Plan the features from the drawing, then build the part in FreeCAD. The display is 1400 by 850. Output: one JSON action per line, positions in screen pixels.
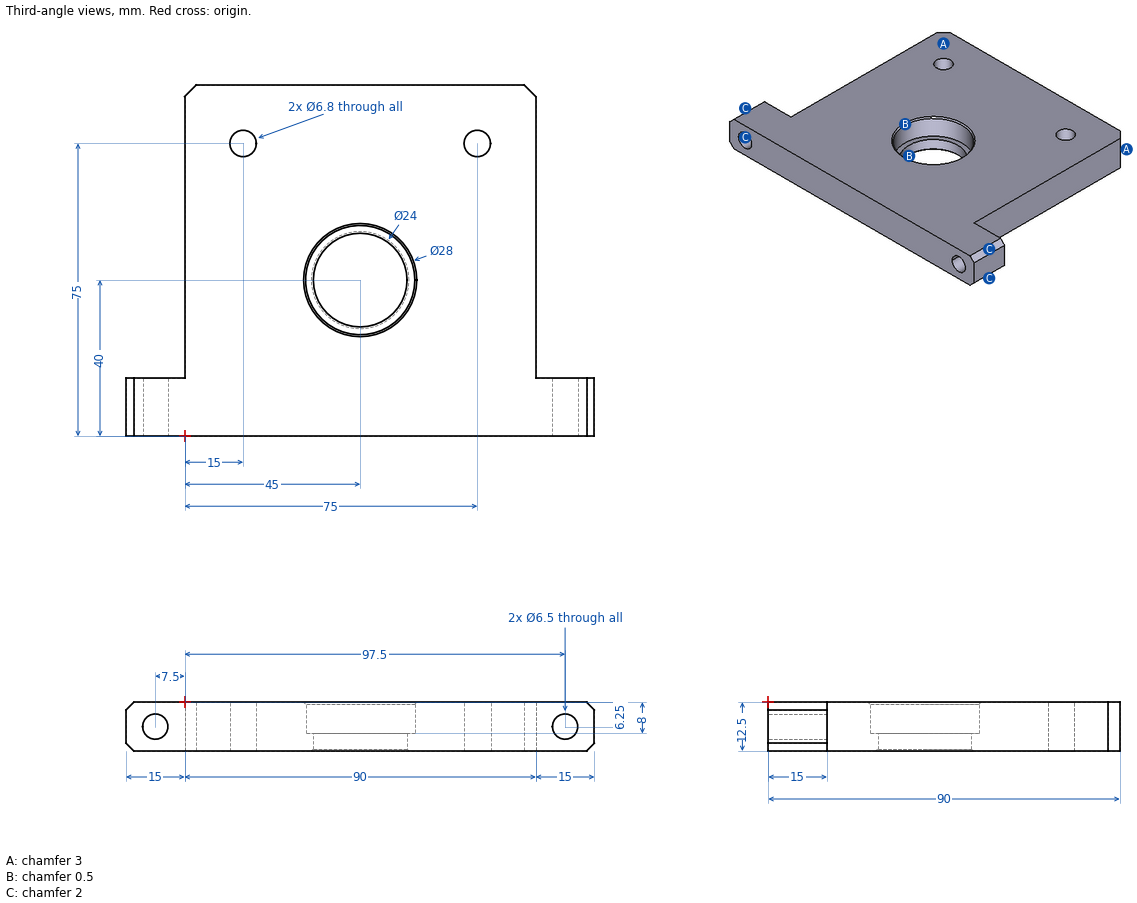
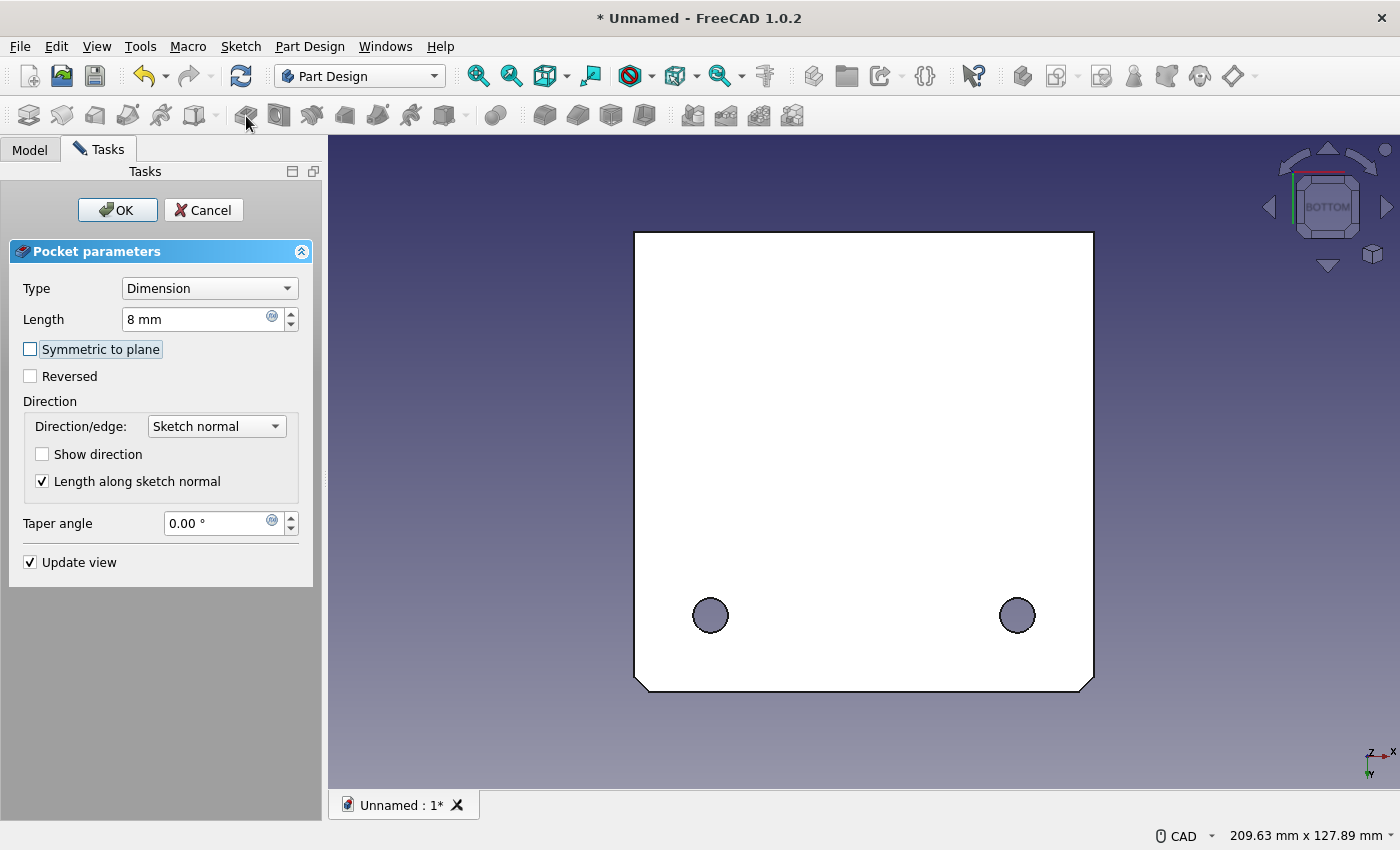
{"action": "left_click", "coordinate": [118, 210]}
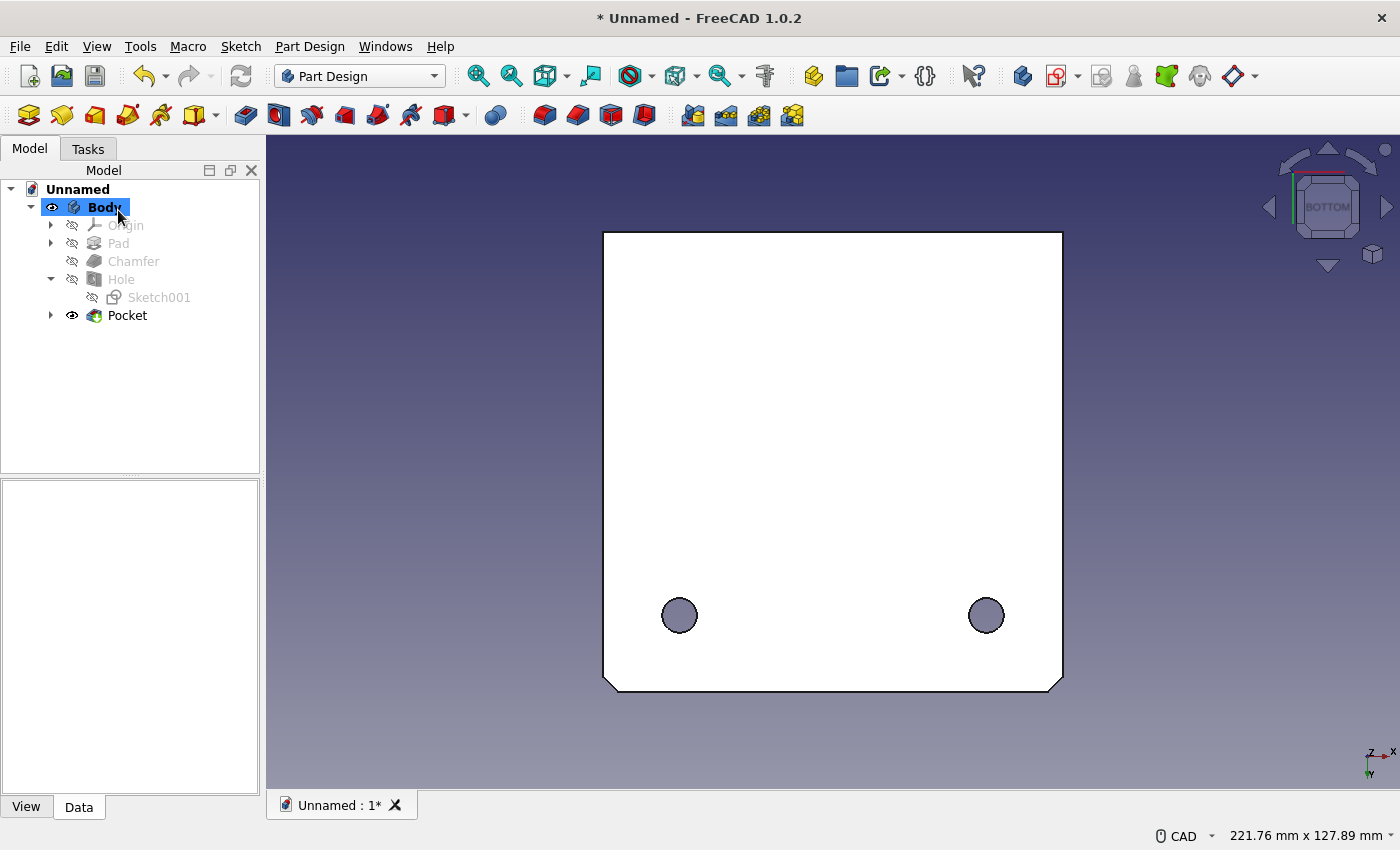
{"action": "key", "text": "0"}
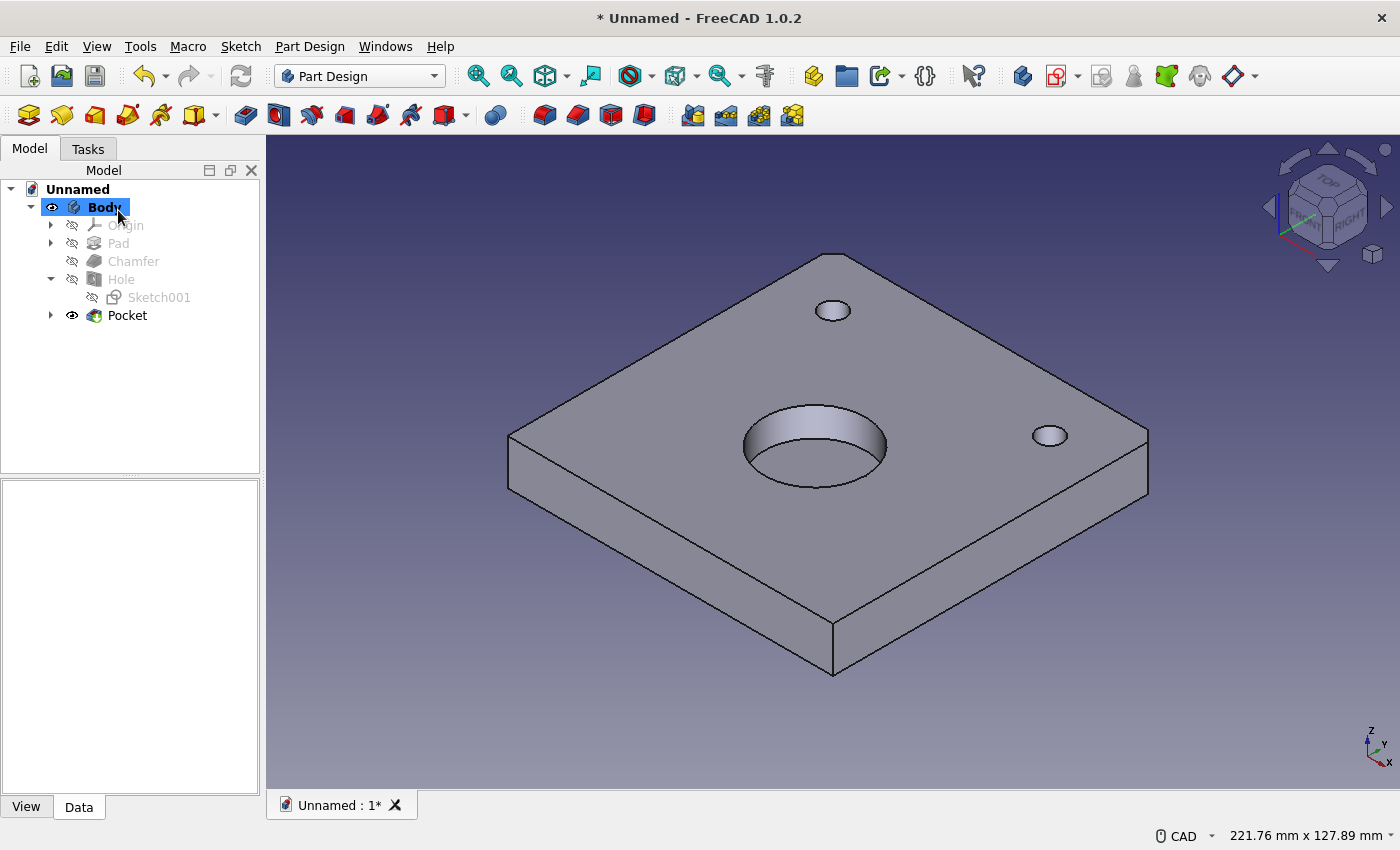
{"action": "left_click", "coordinate": [829, 470]}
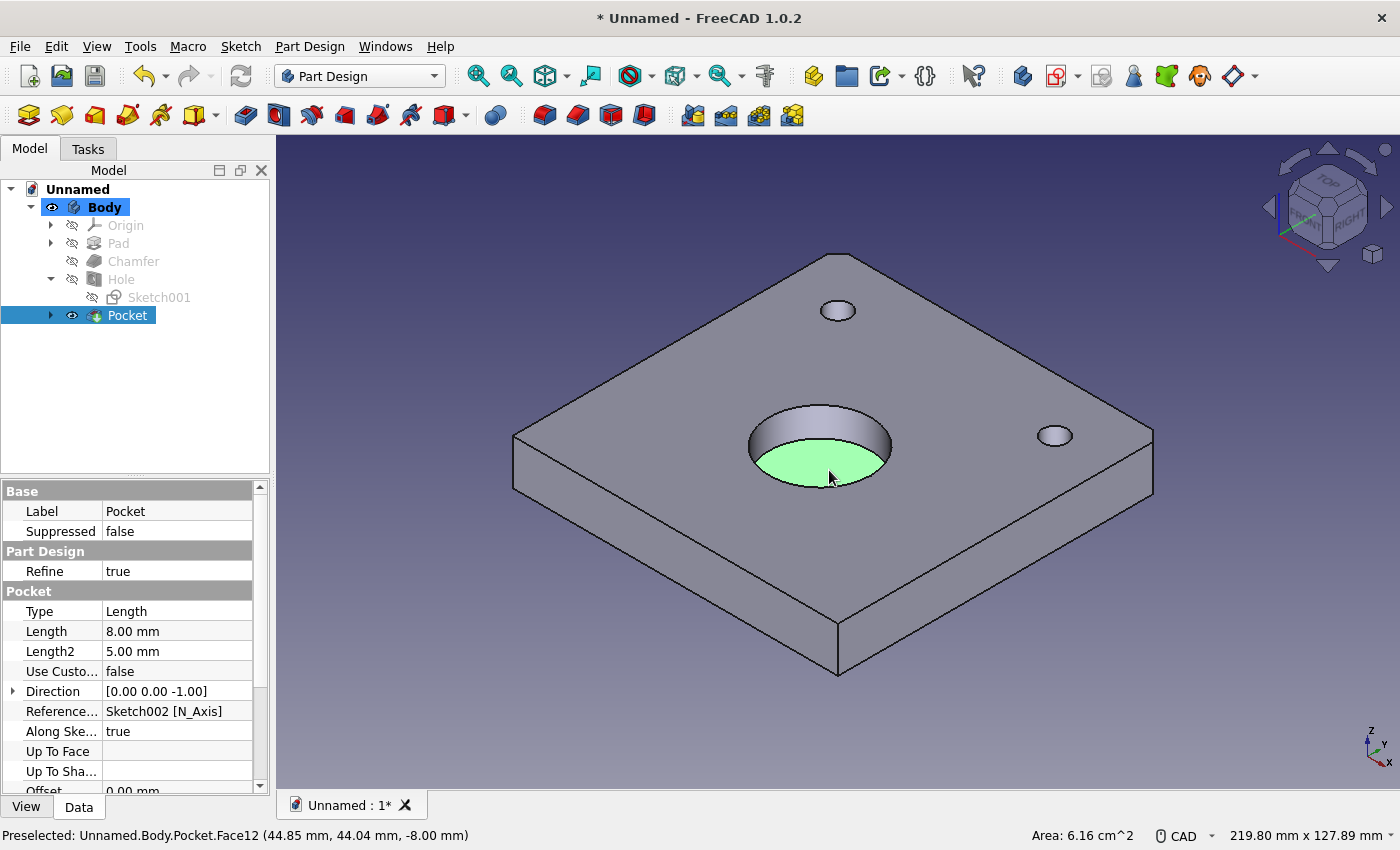
{"action": "left_click", "coordinate": [1056, 76]}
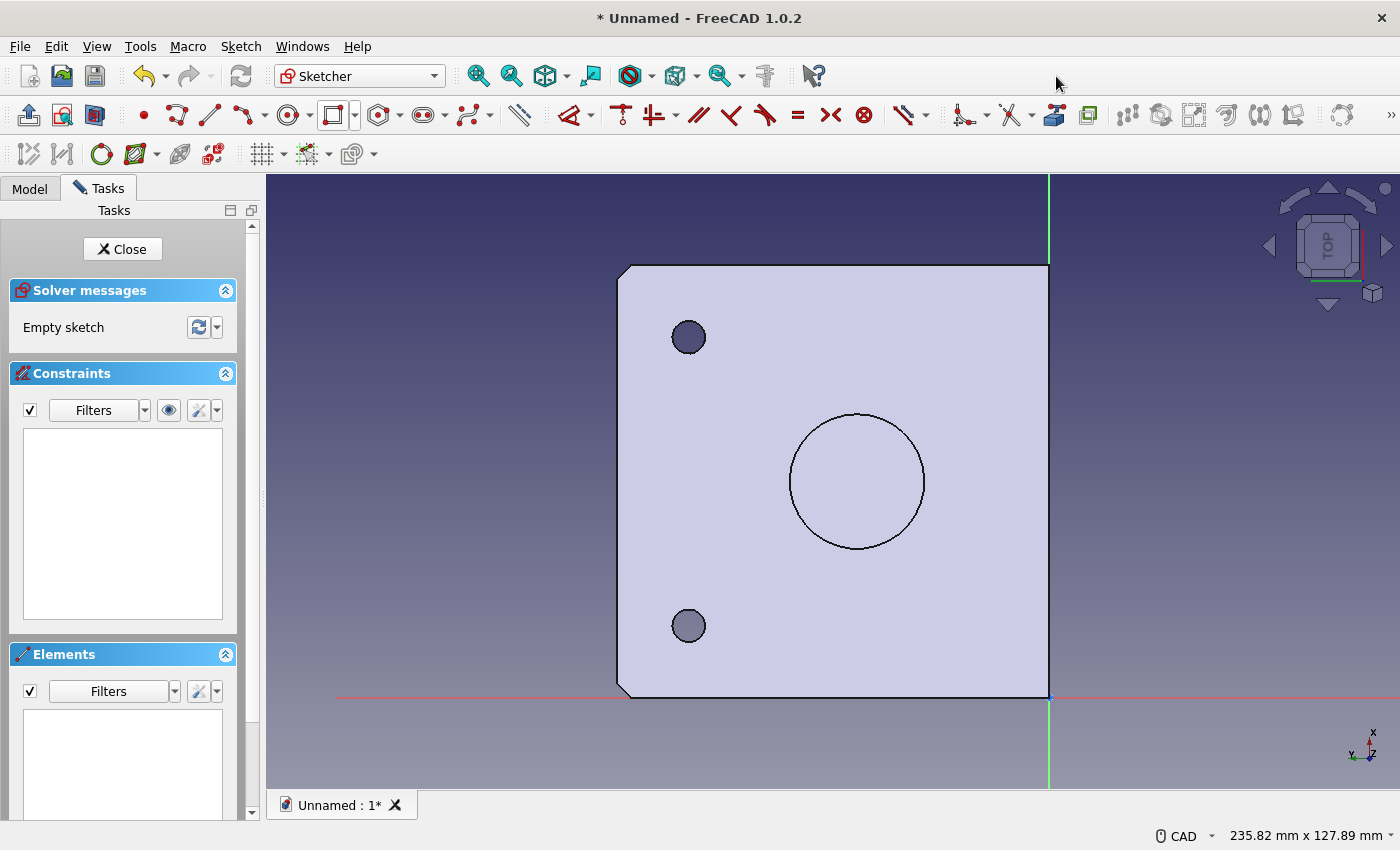
{"action": "left_click", "coordinate": [95, 116]}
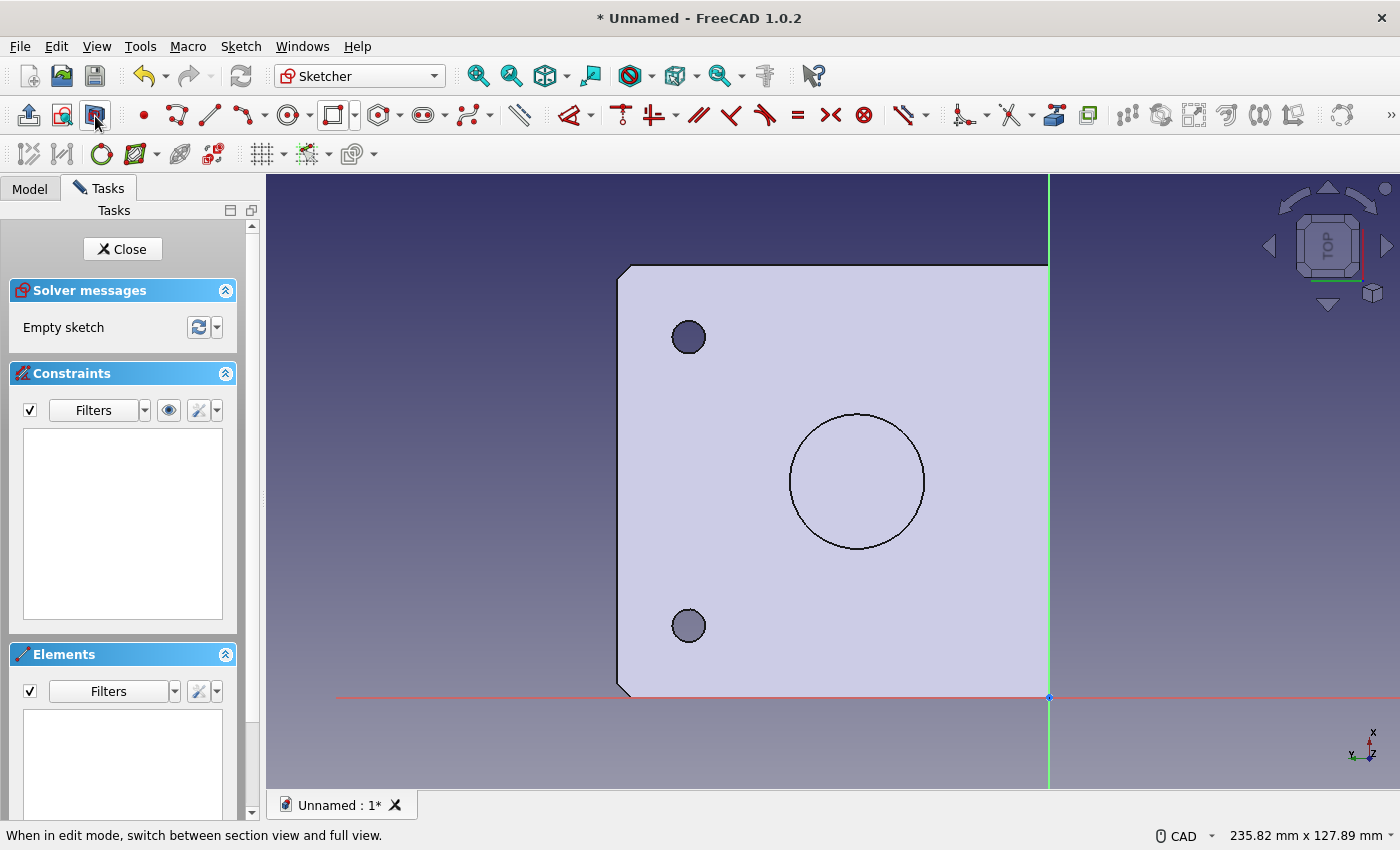
{"action": "scroll", "coordinate": [1235, 722], "scroll_direction": "up", "scroll_amount": 2}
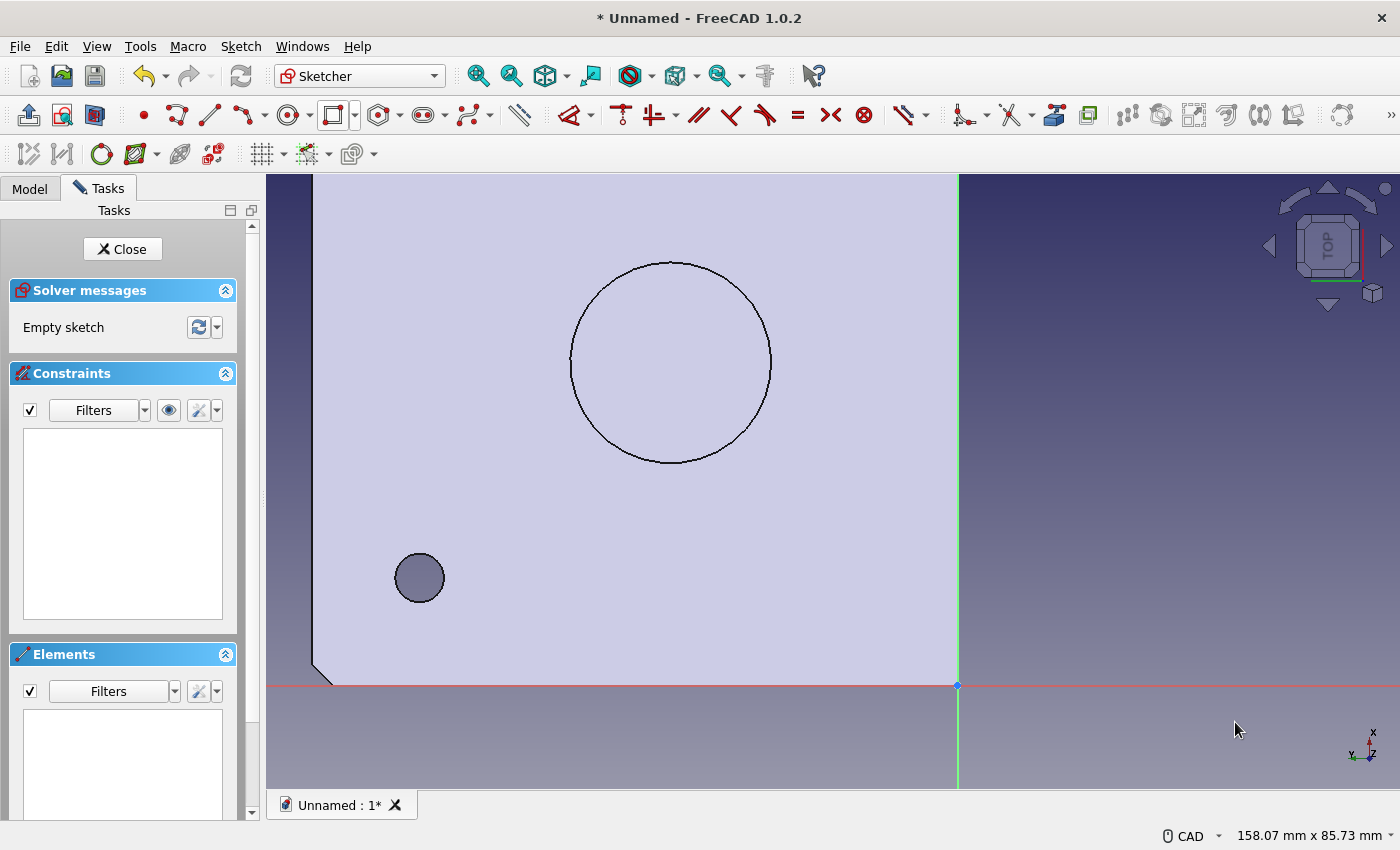
{"action": "left_click", "coordinate": [288, 116]}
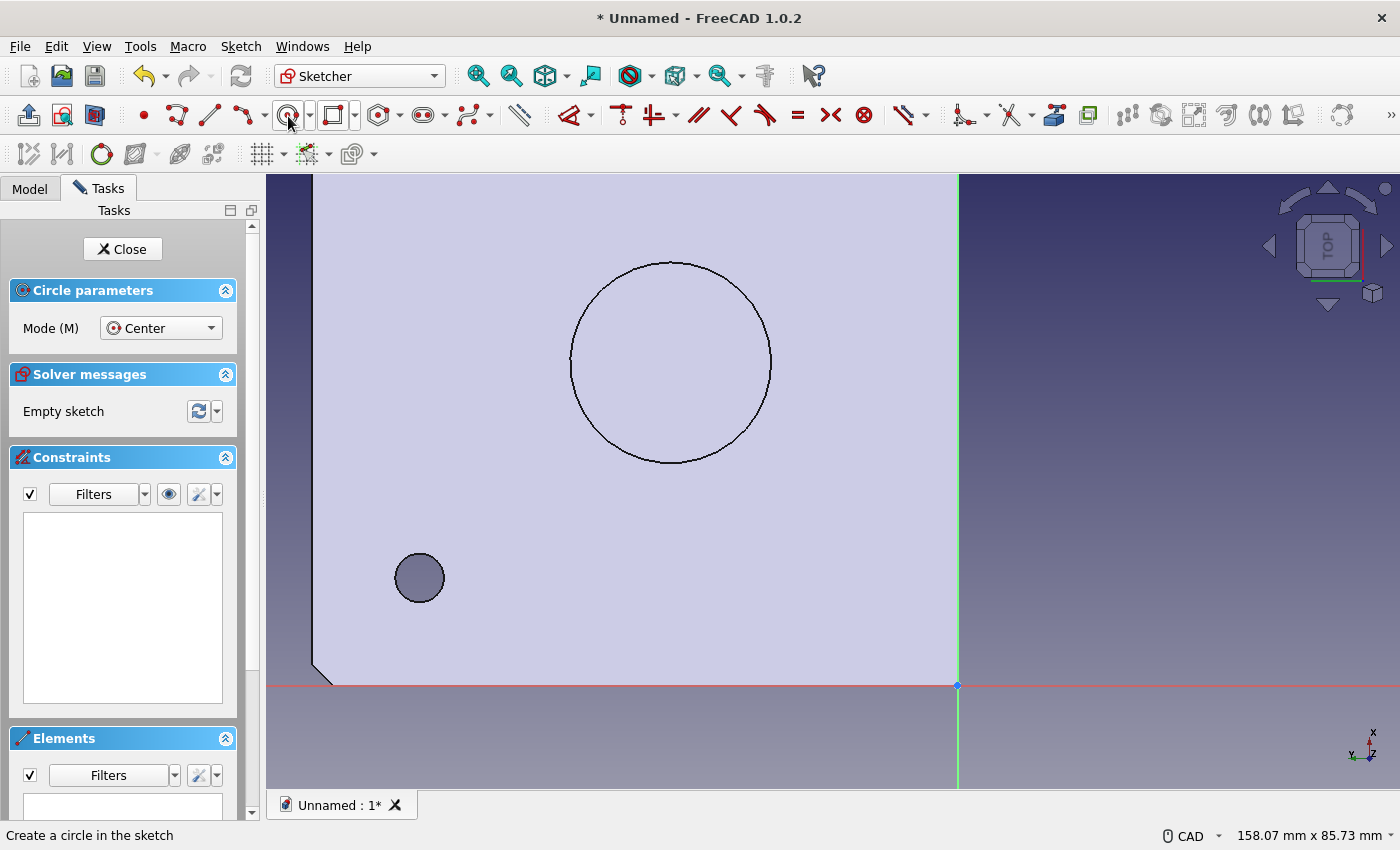
{"action": "left_click", "coordinate": [671, 363]}
{"action": "left_click", "coordinate": [732, 302]}
{"action": "key", "text": "Escape"}